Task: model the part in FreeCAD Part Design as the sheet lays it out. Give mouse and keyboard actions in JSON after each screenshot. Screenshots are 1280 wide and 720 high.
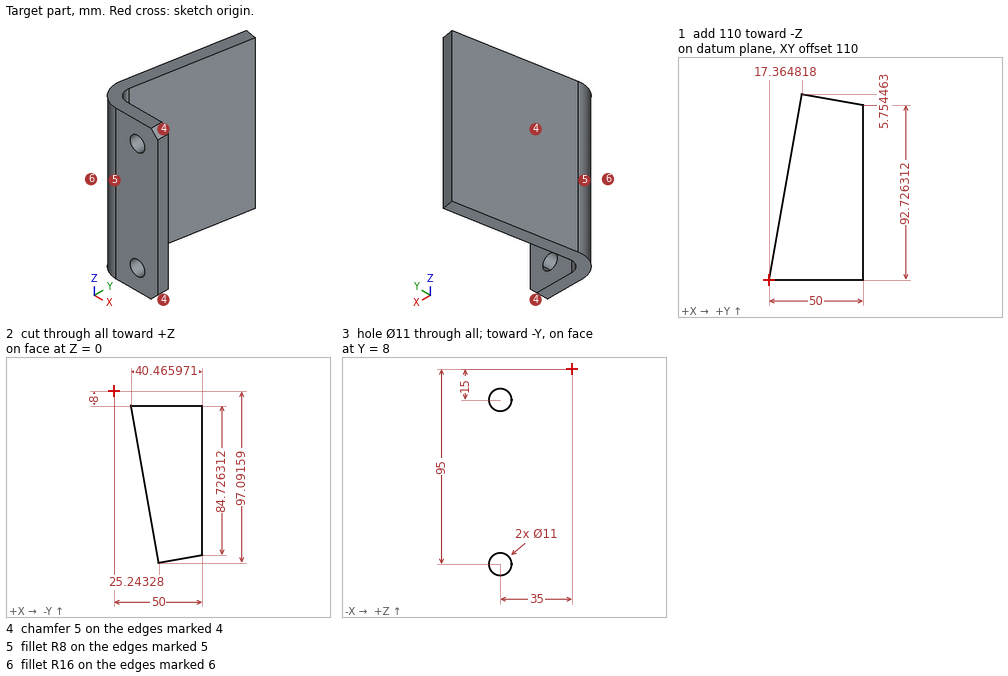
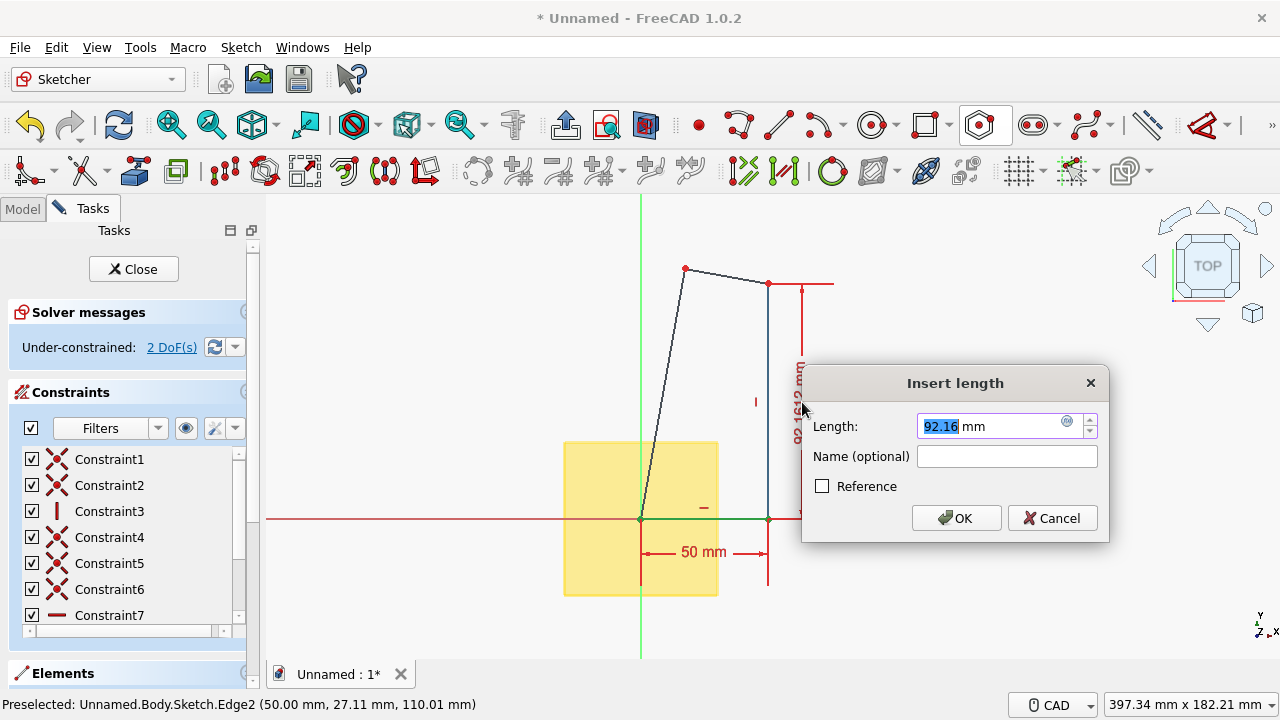
{"action": "type", "text": "92.726312"}
{"action": "key", "text": "Return"}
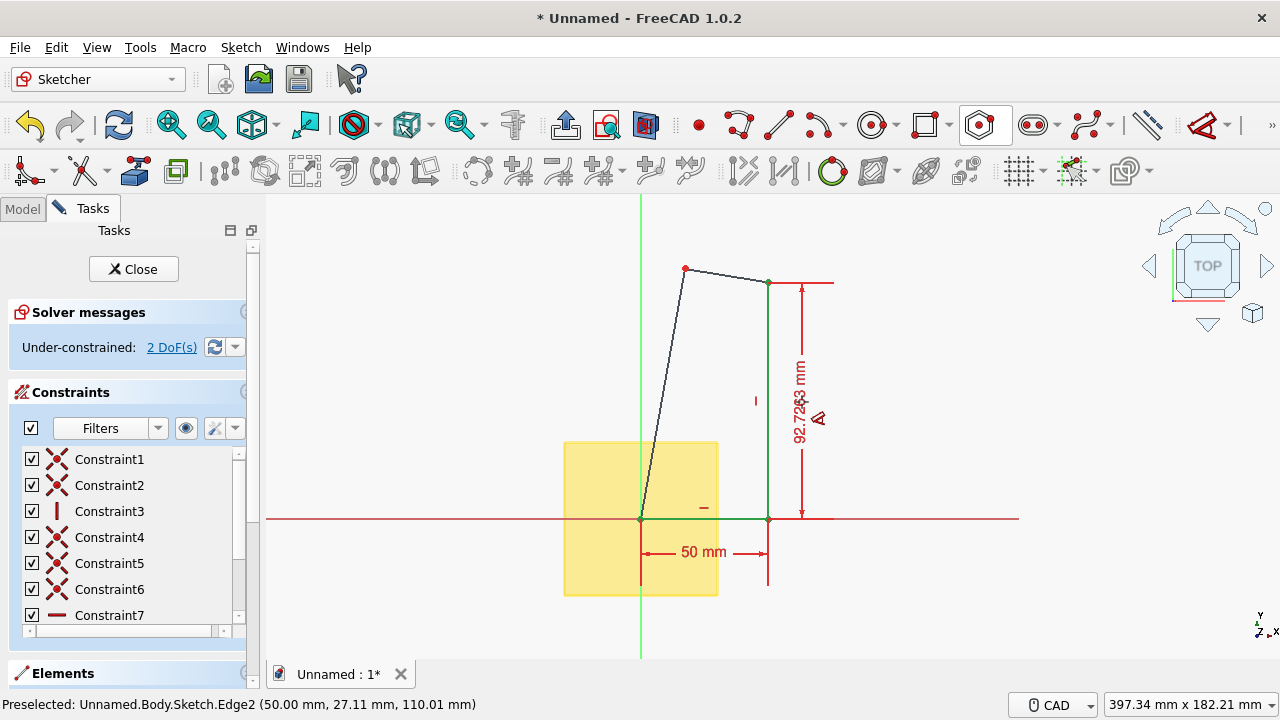
{"action": "scroll", "coordinate": [743, 278], "scroll_direction": "up", "scroll_amount": 5}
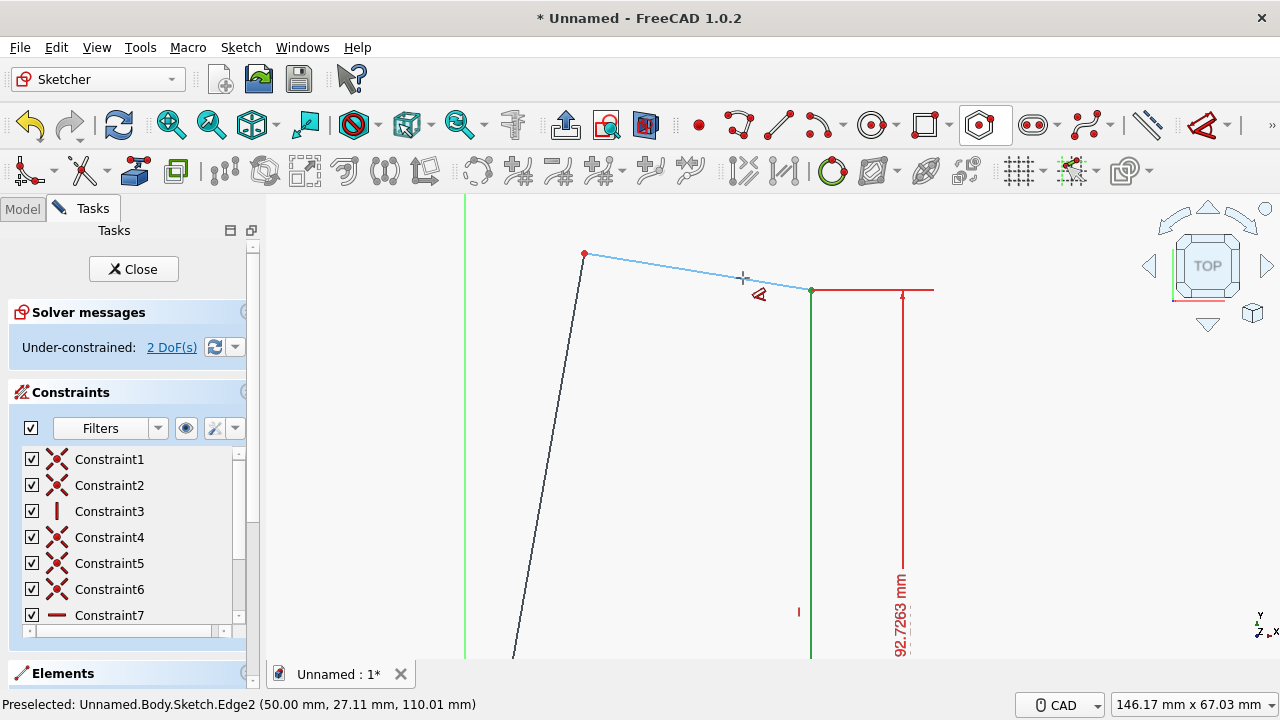
{"action": "left_click", "coordinate": [743, 279]}
{"action": "left_click", "coordinate": [845, 272]}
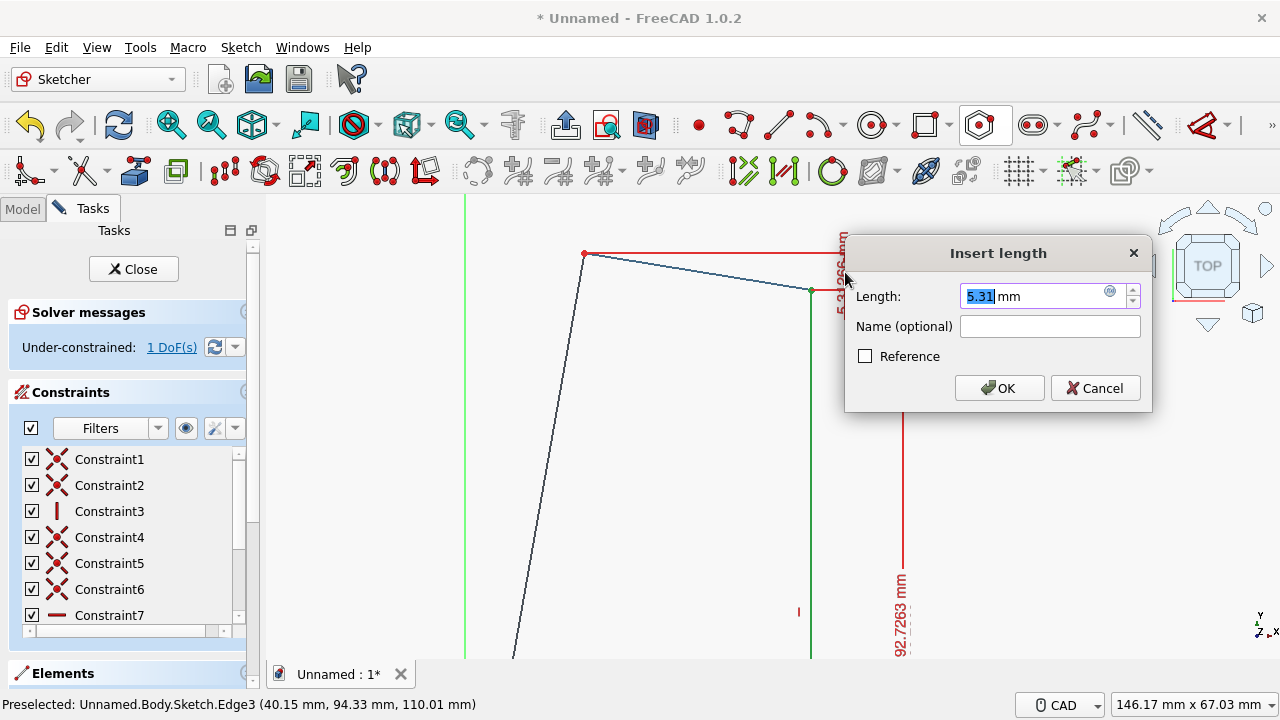
{"action": "type", "text": "5.754463"}
{"action": "key", "text": "Return"}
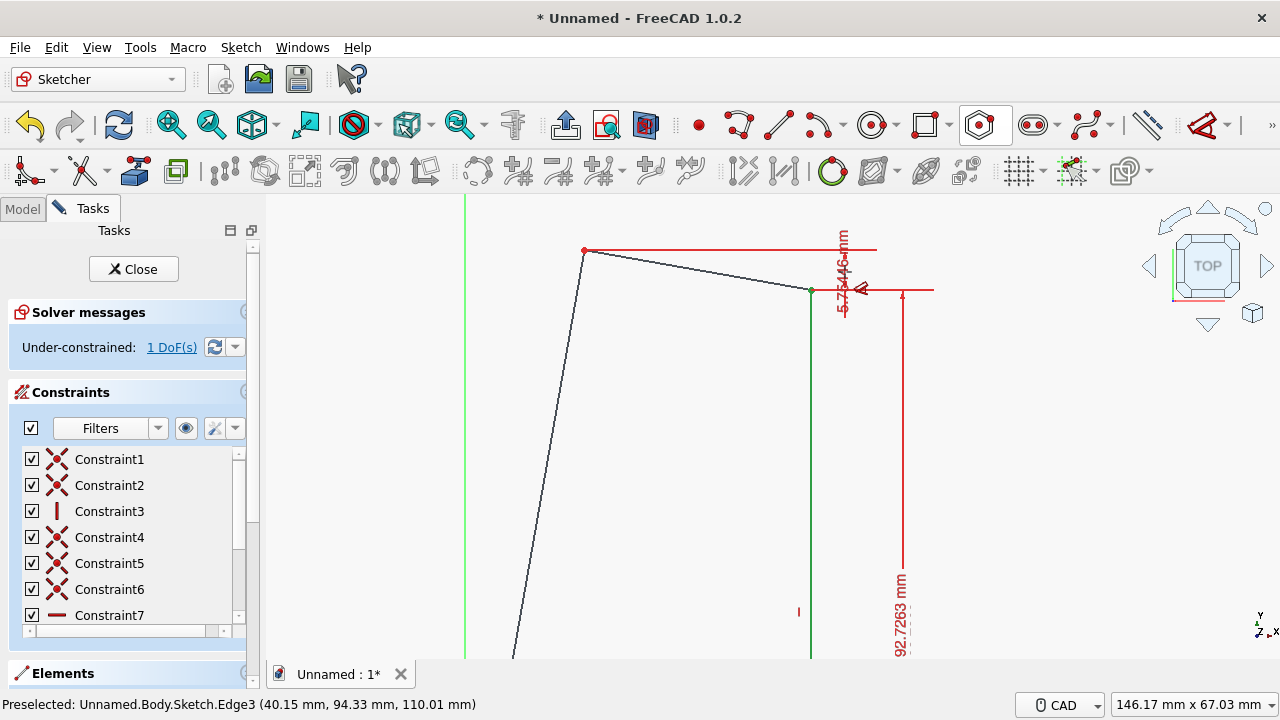
{"action": "left_click", "coordinate": [585, 250]}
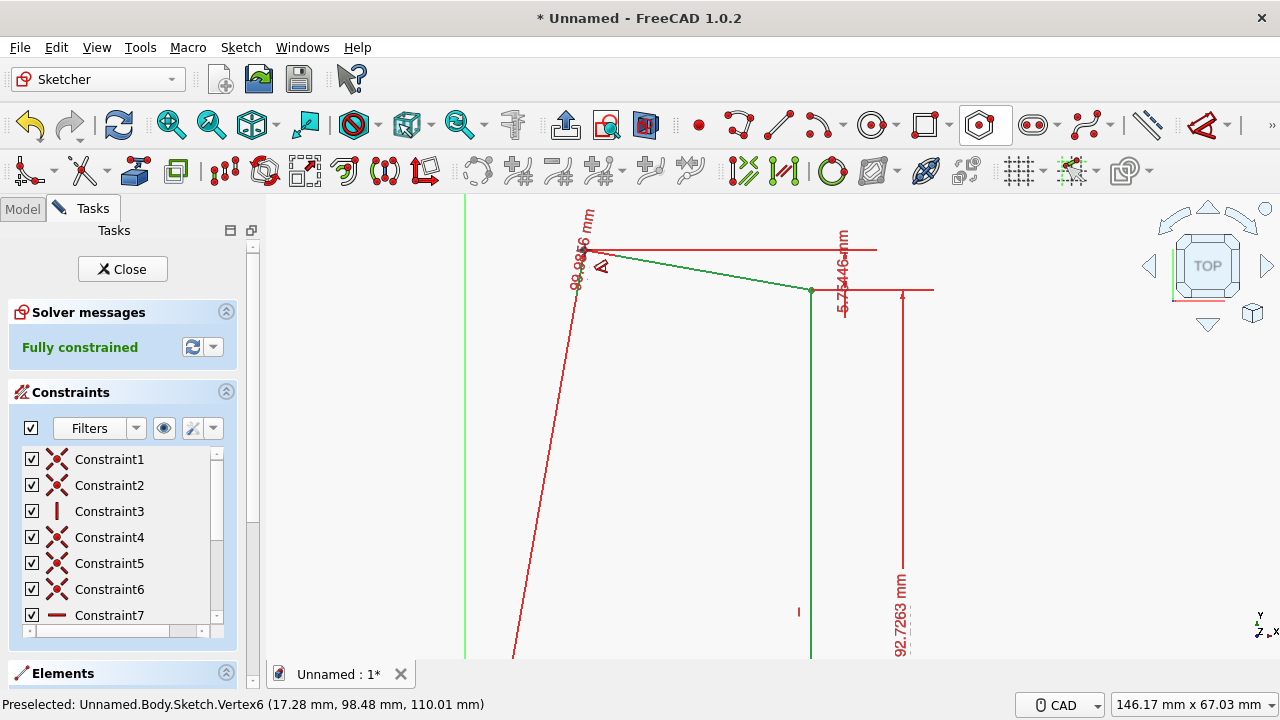
{"action": "key", "text": "Escape"}
{"action": "key", "text": "Escape"}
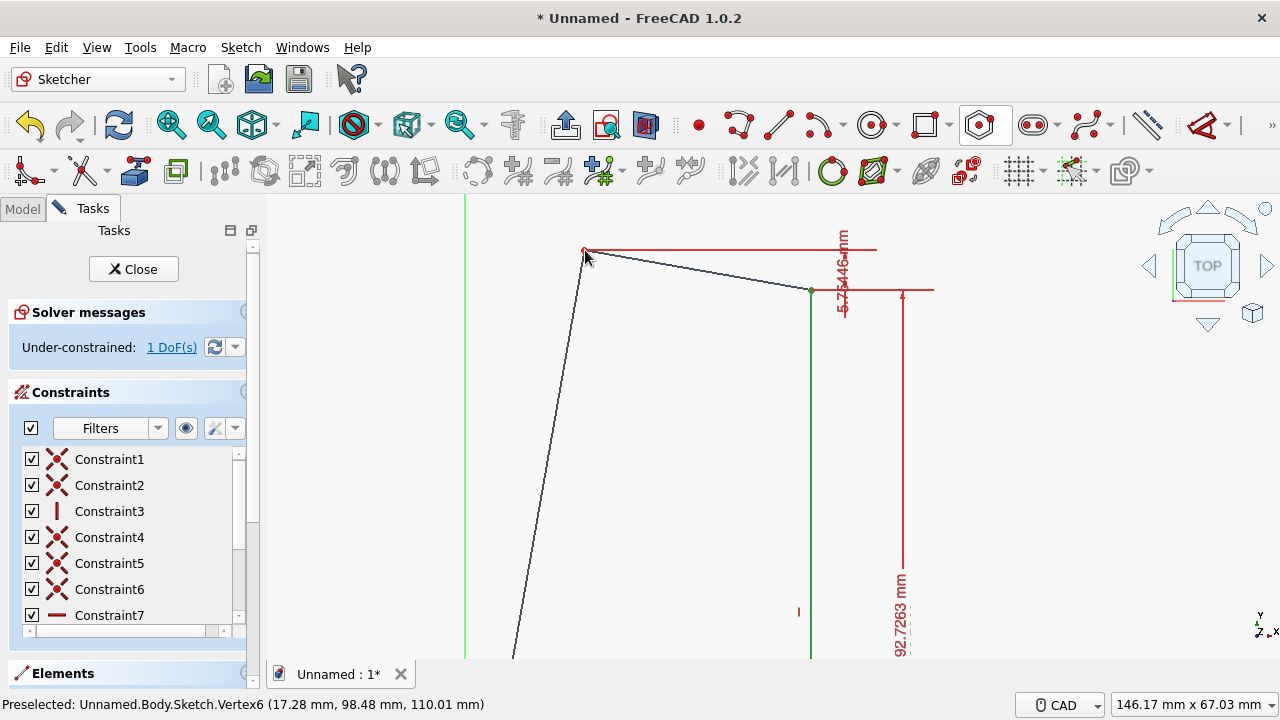
{"action": "left_click", "coordinate": [585, 250]}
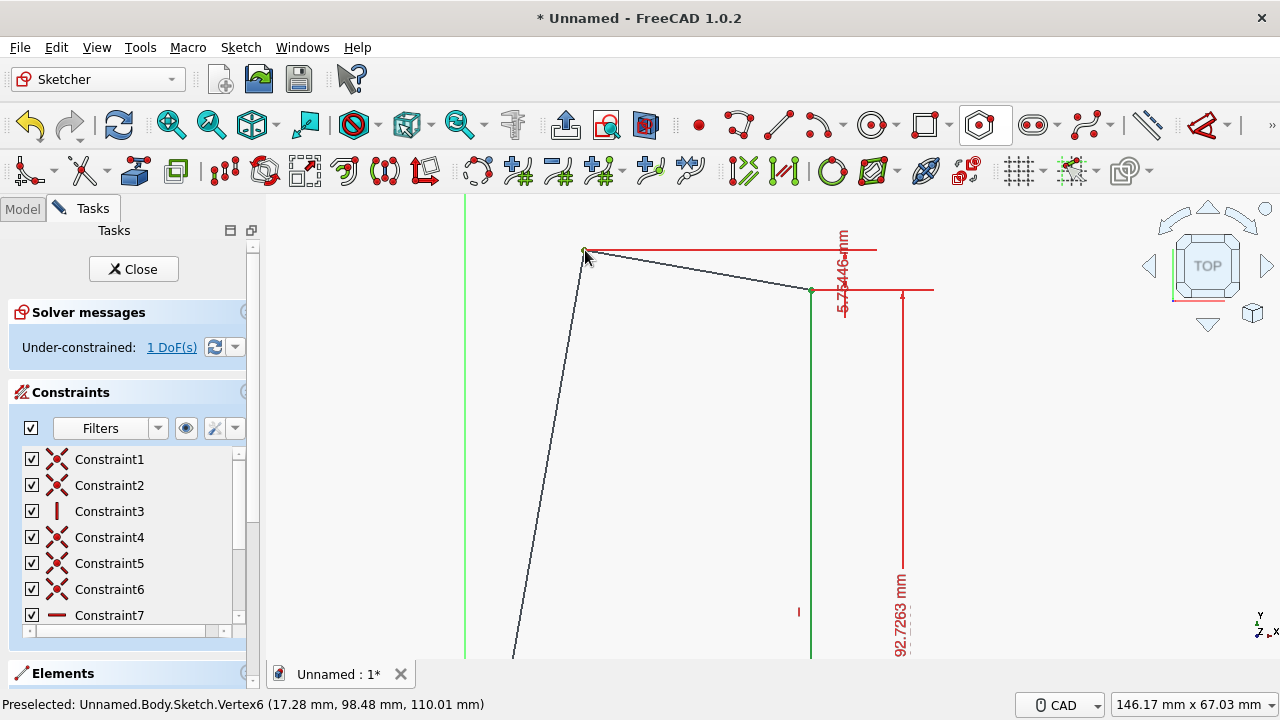
{"action": "key", "text": "l"}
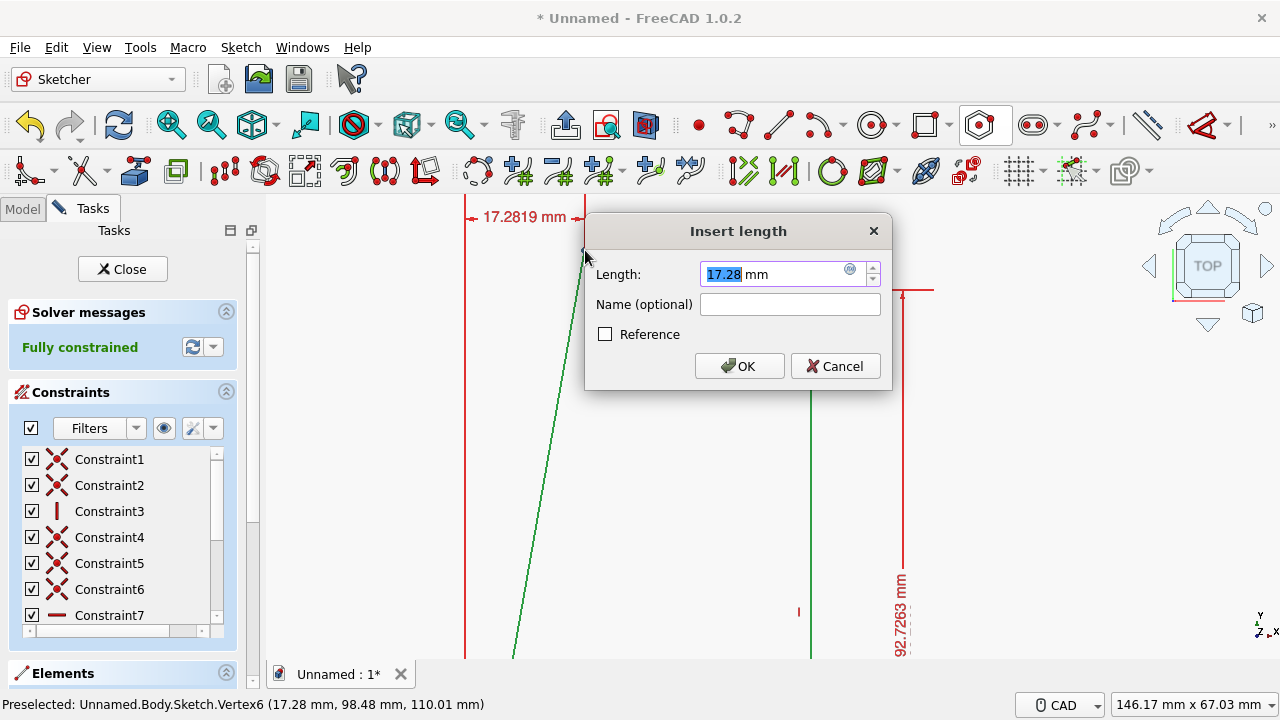
{"action": "type", "text": "17.364818"}
{"action": "key", "text": "Return"}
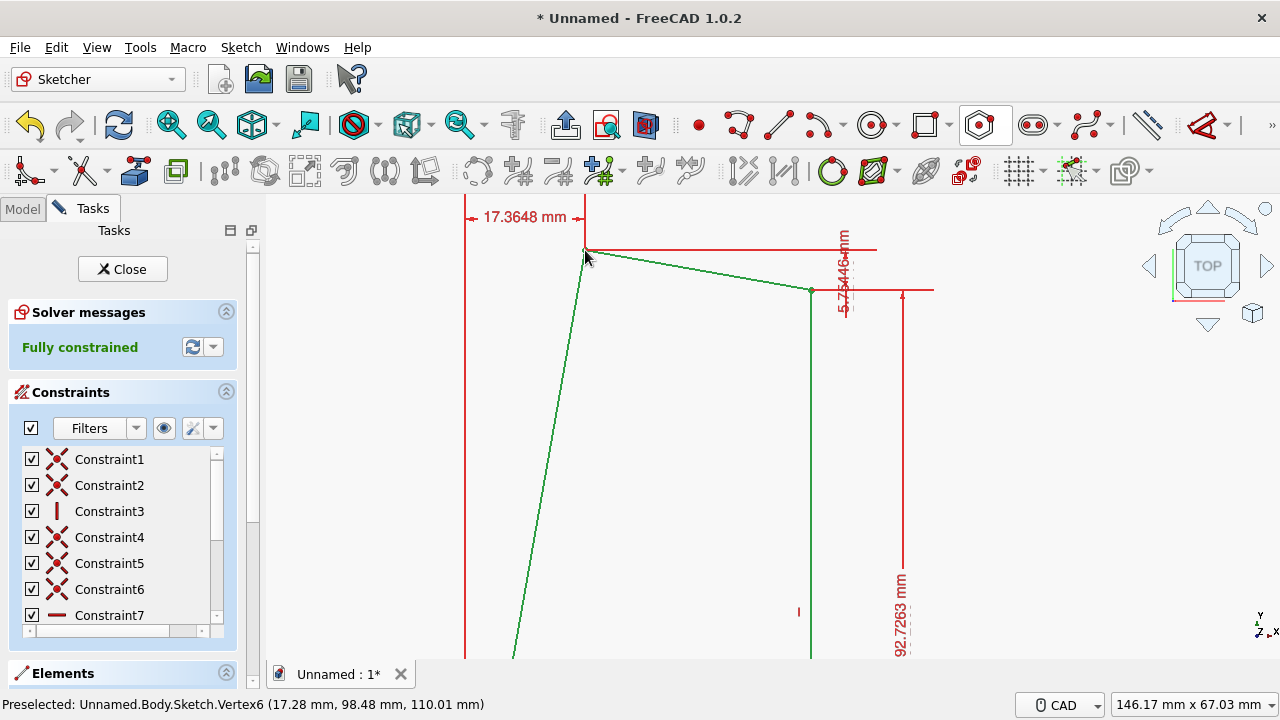
{"action": "left_click", "coordinate": [123, 269]}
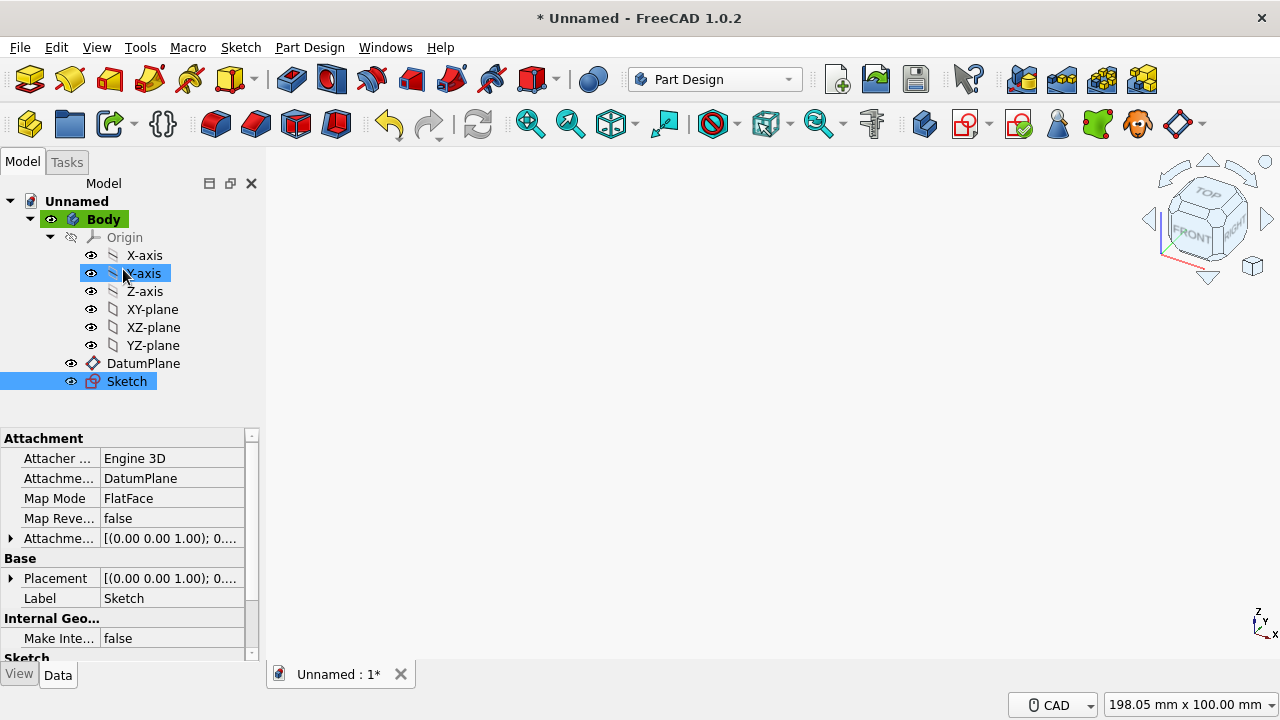
{"action": "left_click", "coordinate": [30, 80]}